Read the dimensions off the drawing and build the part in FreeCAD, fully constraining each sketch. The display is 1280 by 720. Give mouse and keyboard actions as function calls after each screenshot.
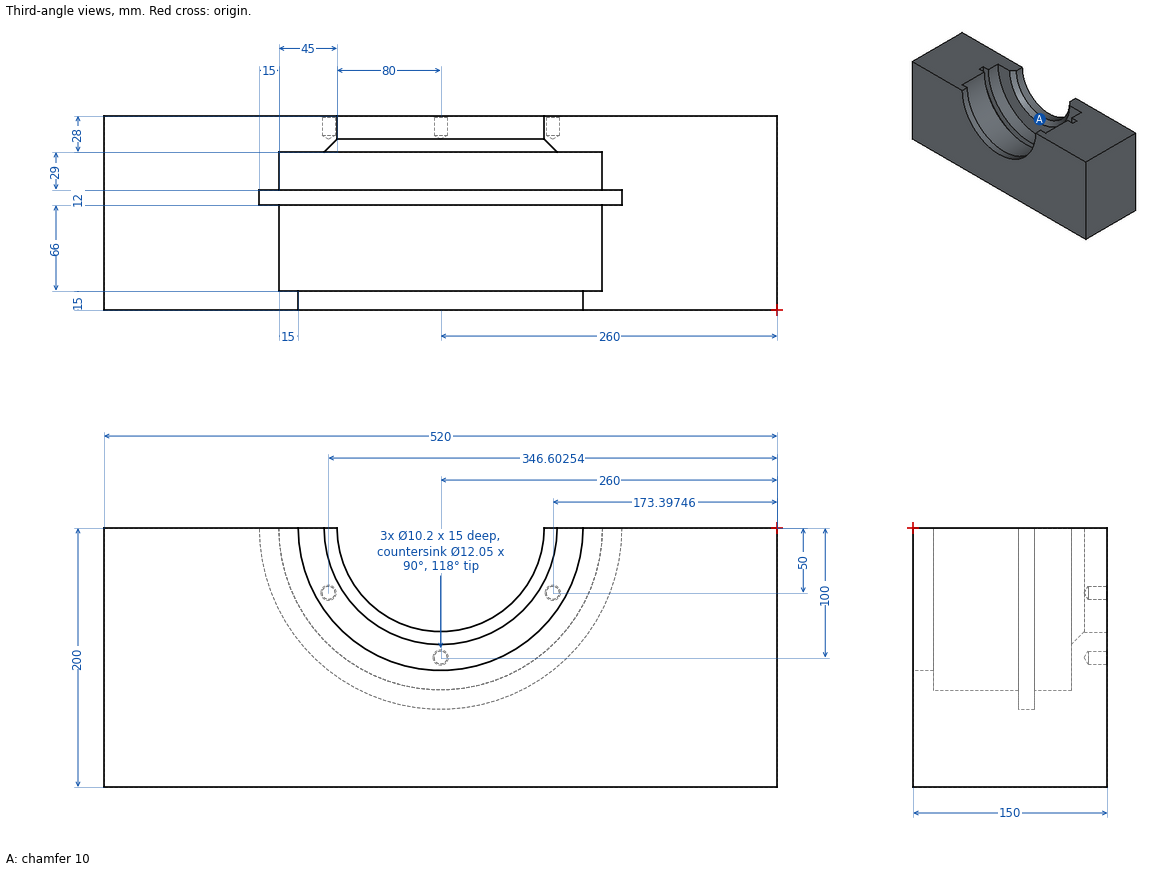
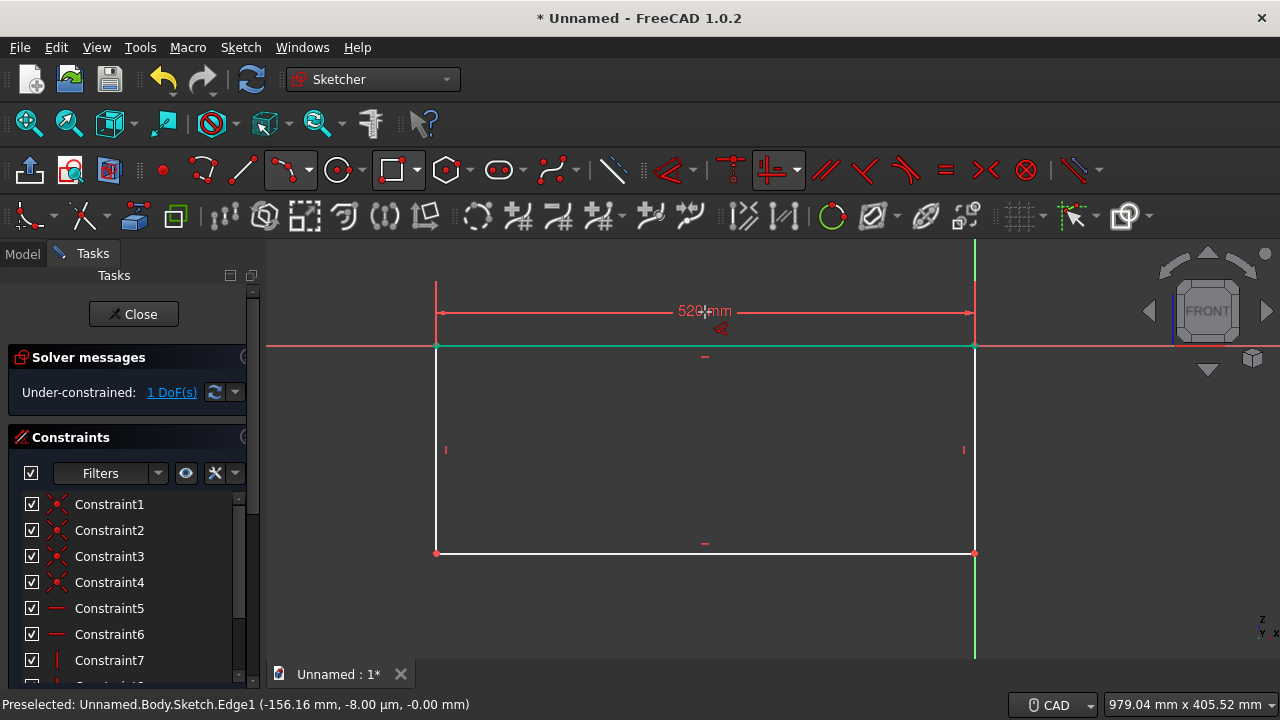
click(436, 408)
click(402, 450)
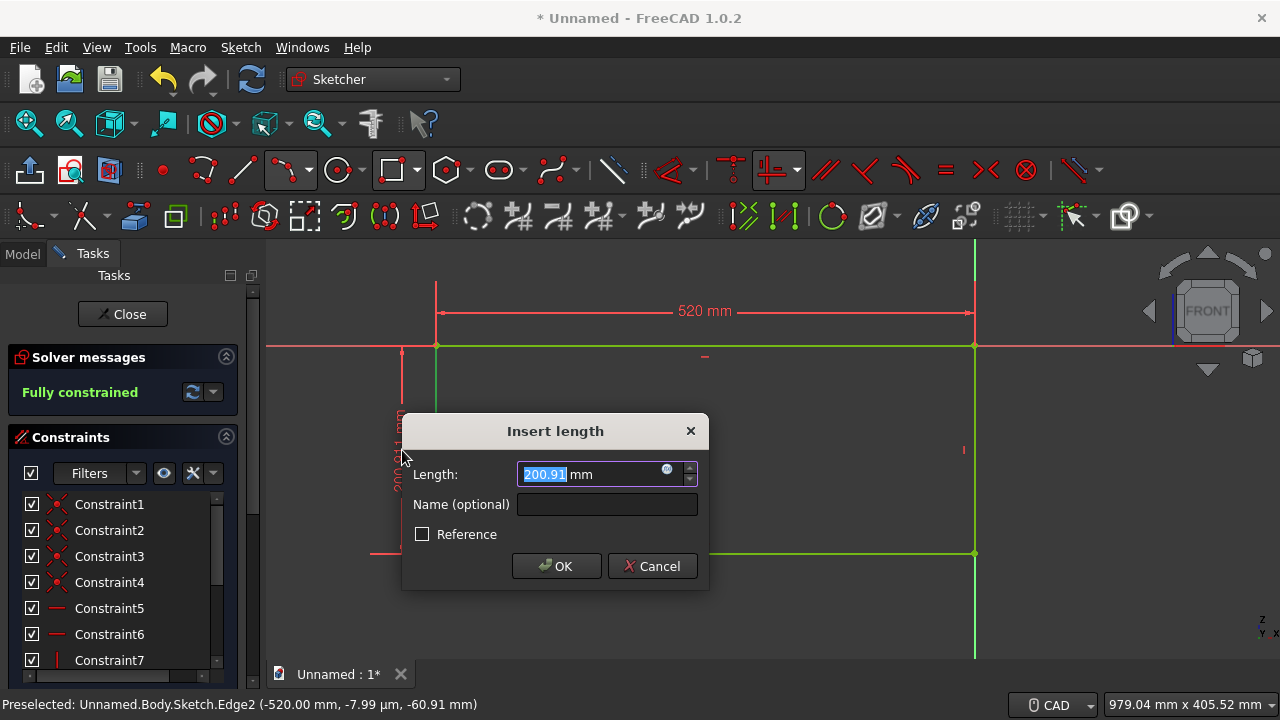
text(200)
key(Return)
key(Escape)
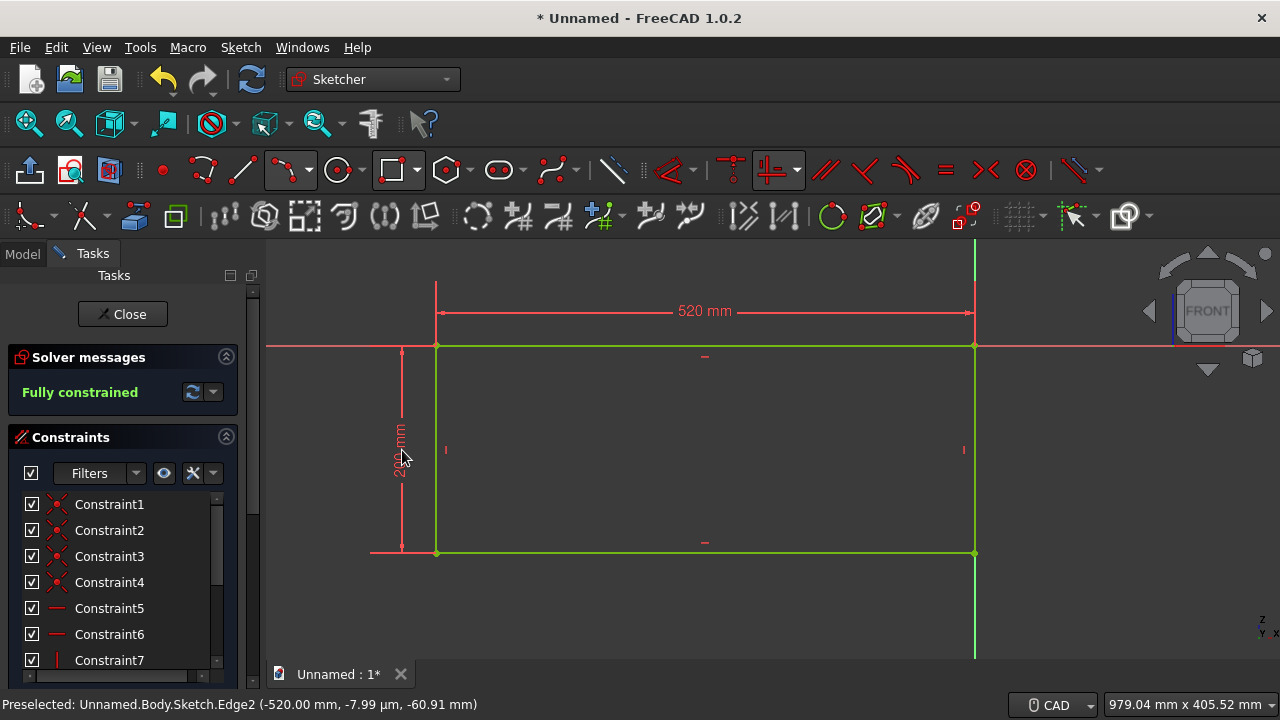
click(123, 314)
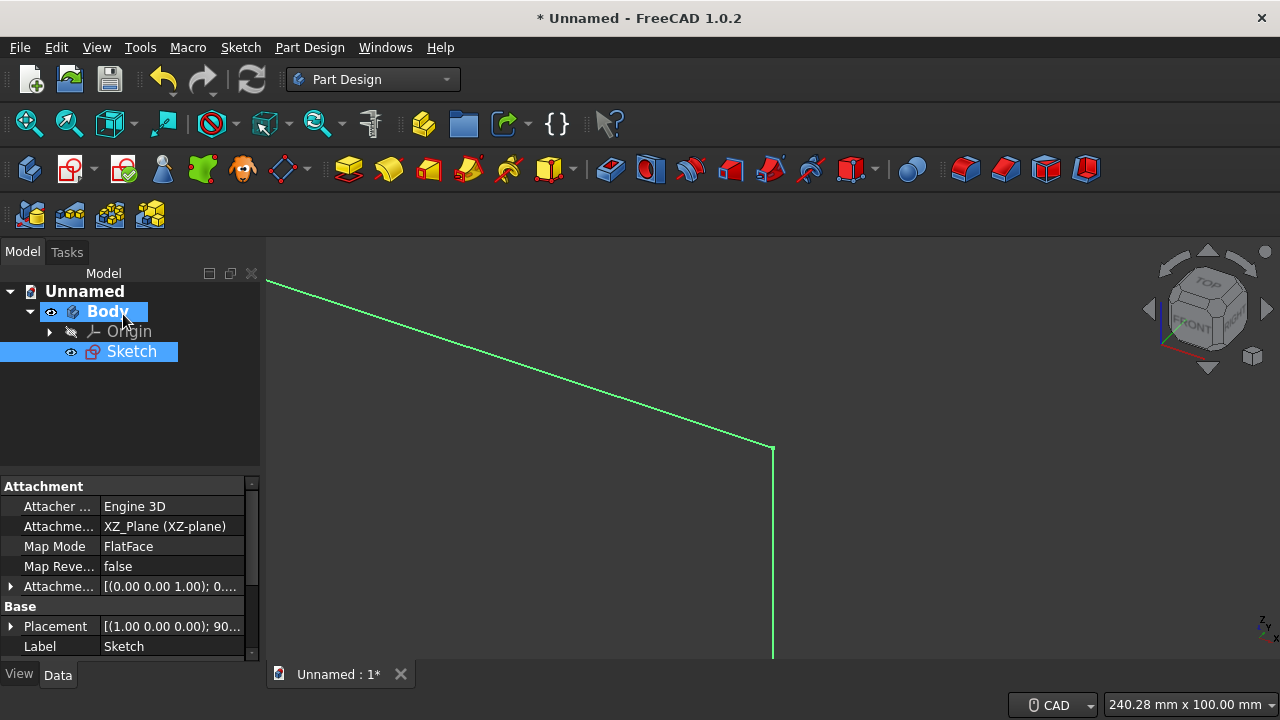
click(350, 170)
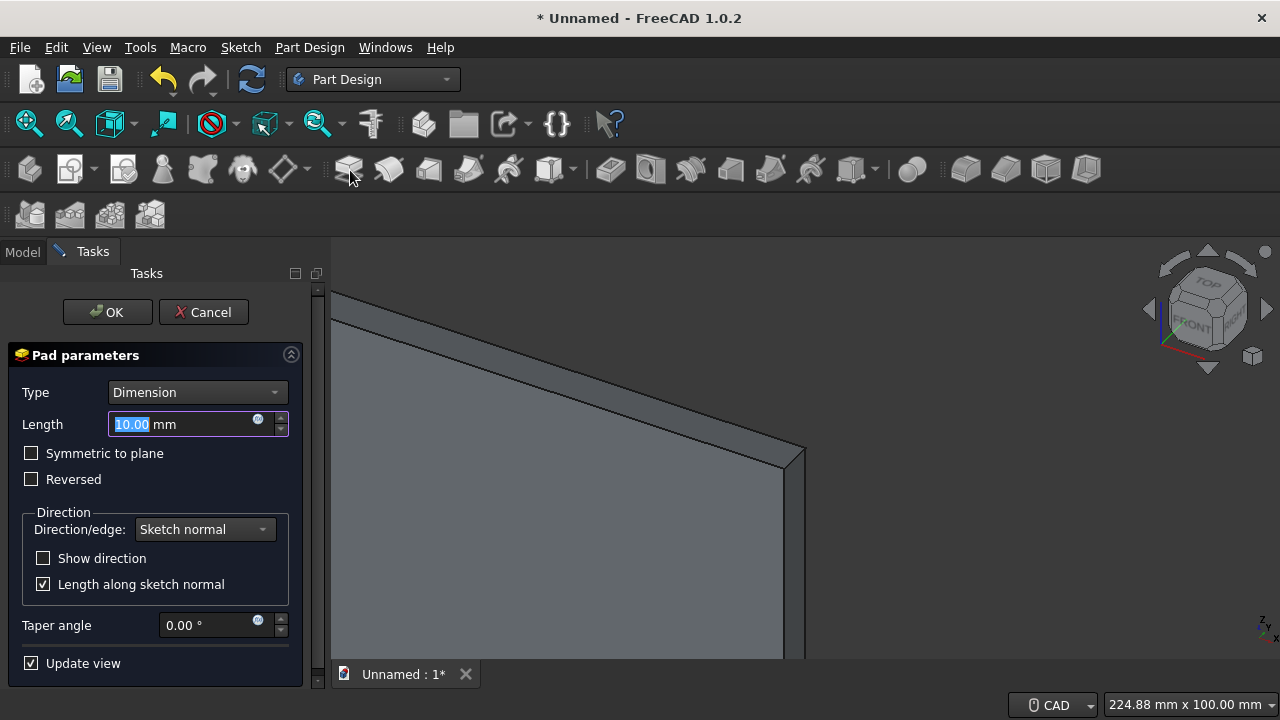
text(150)
key(Tab)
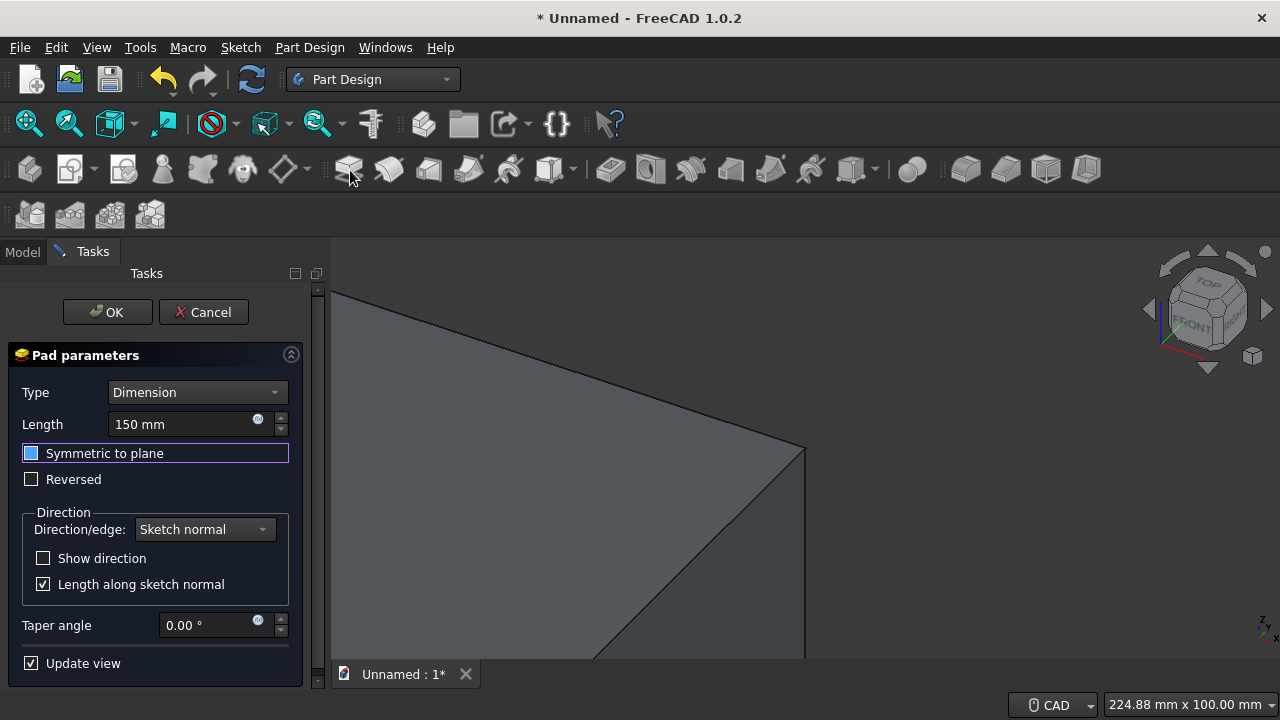
click(30, 479)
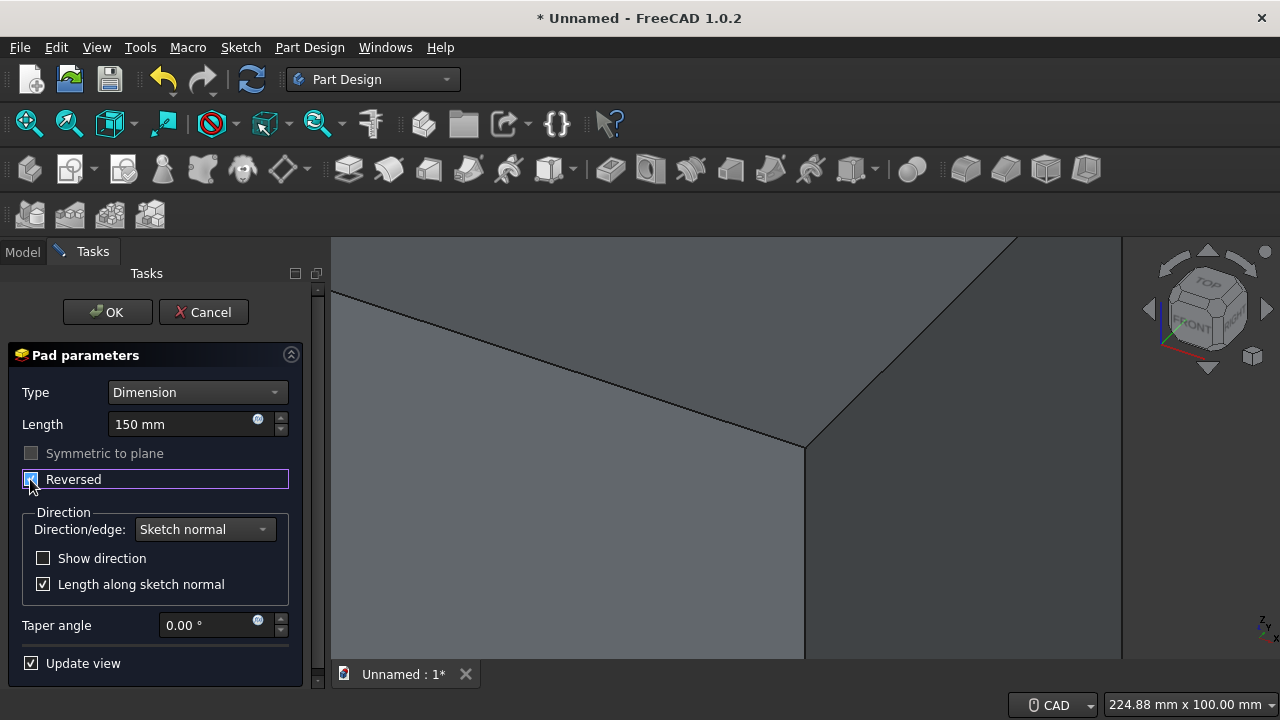
click(108, 312)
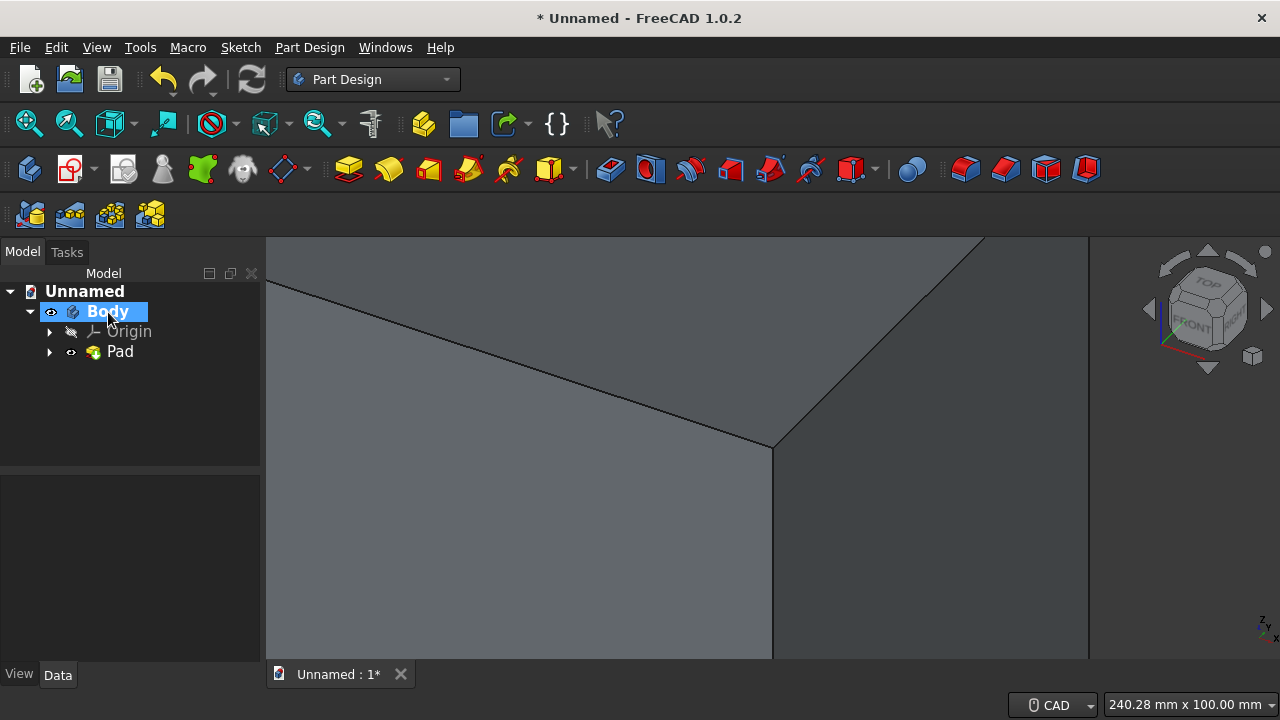
key(v)
key(f)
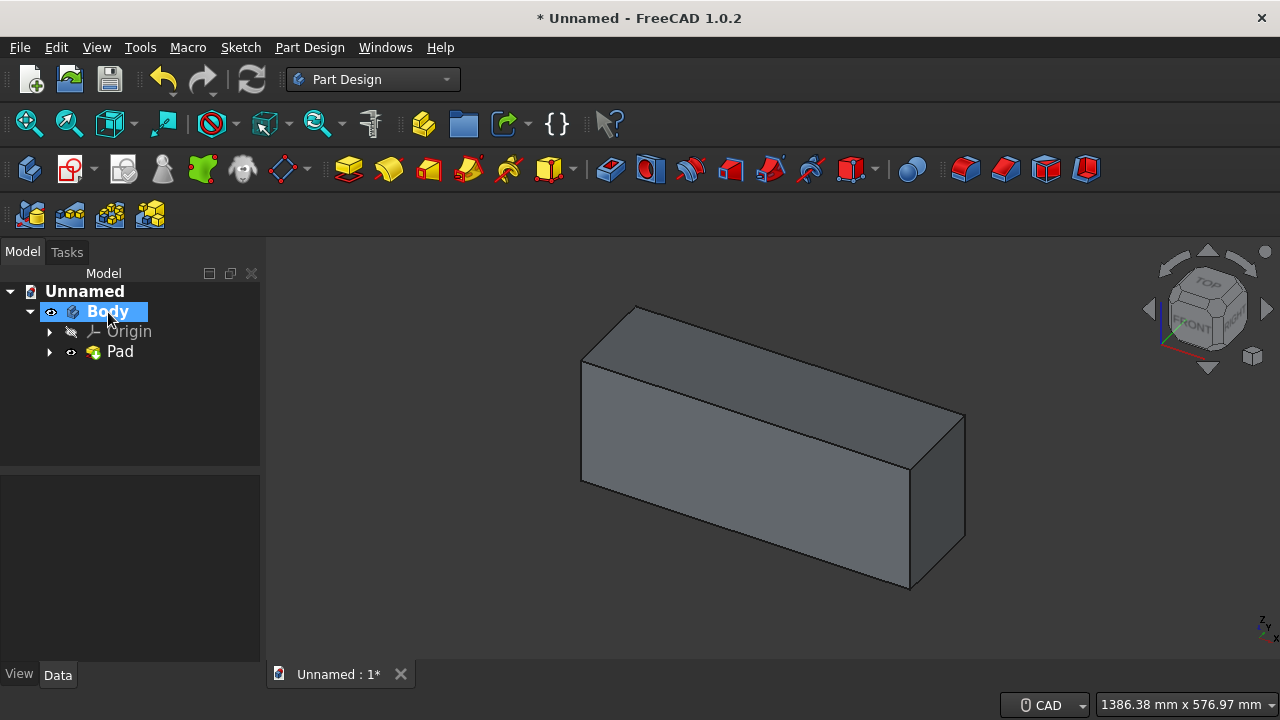
key(4)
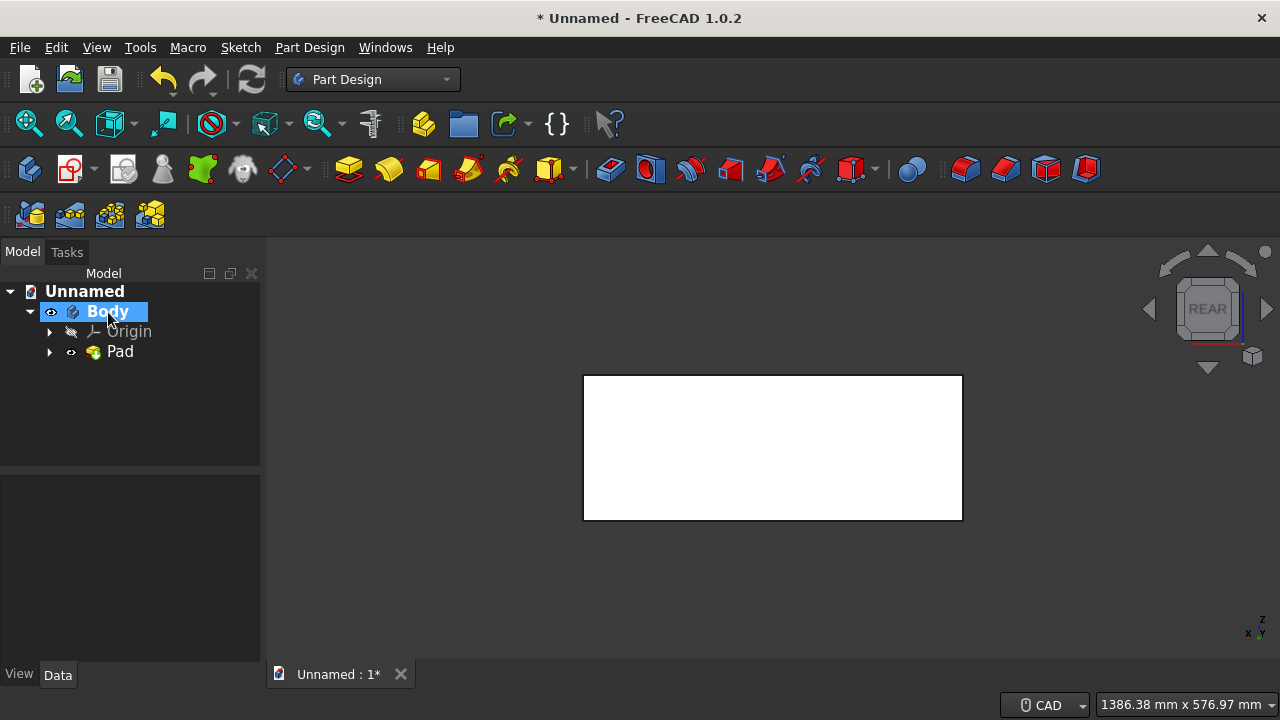
click(30, 124)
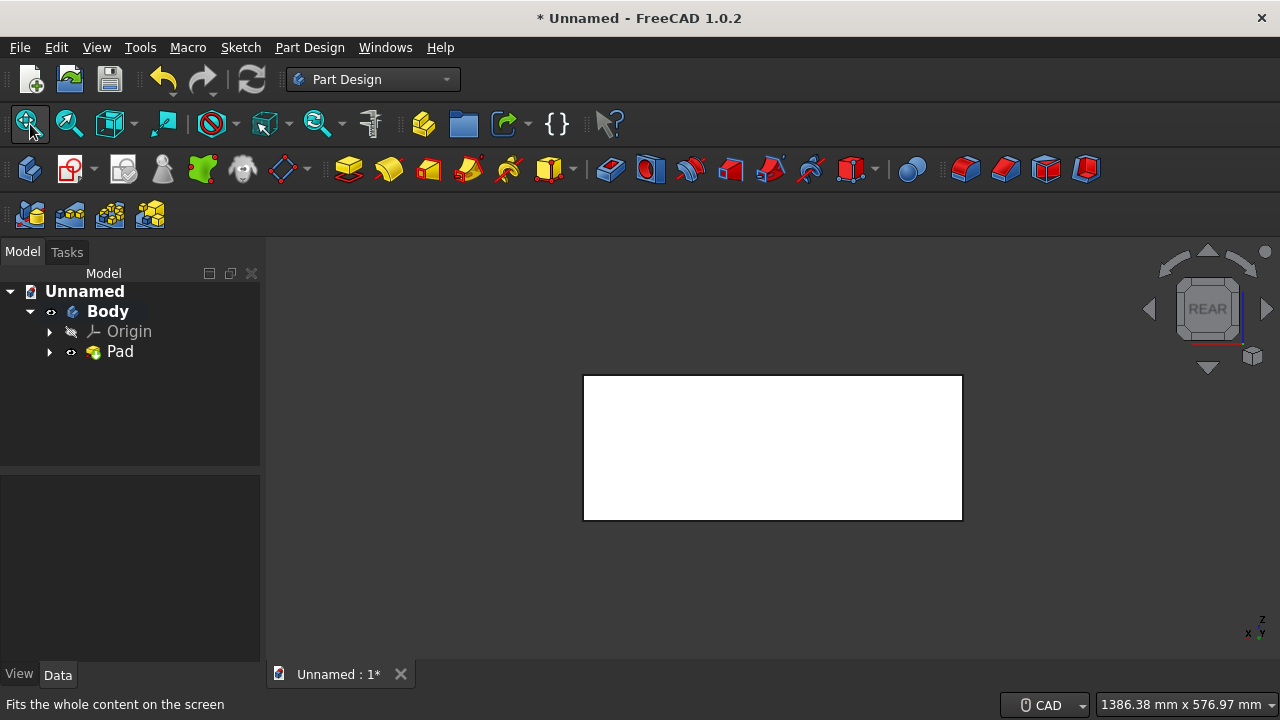
click(664, 447)